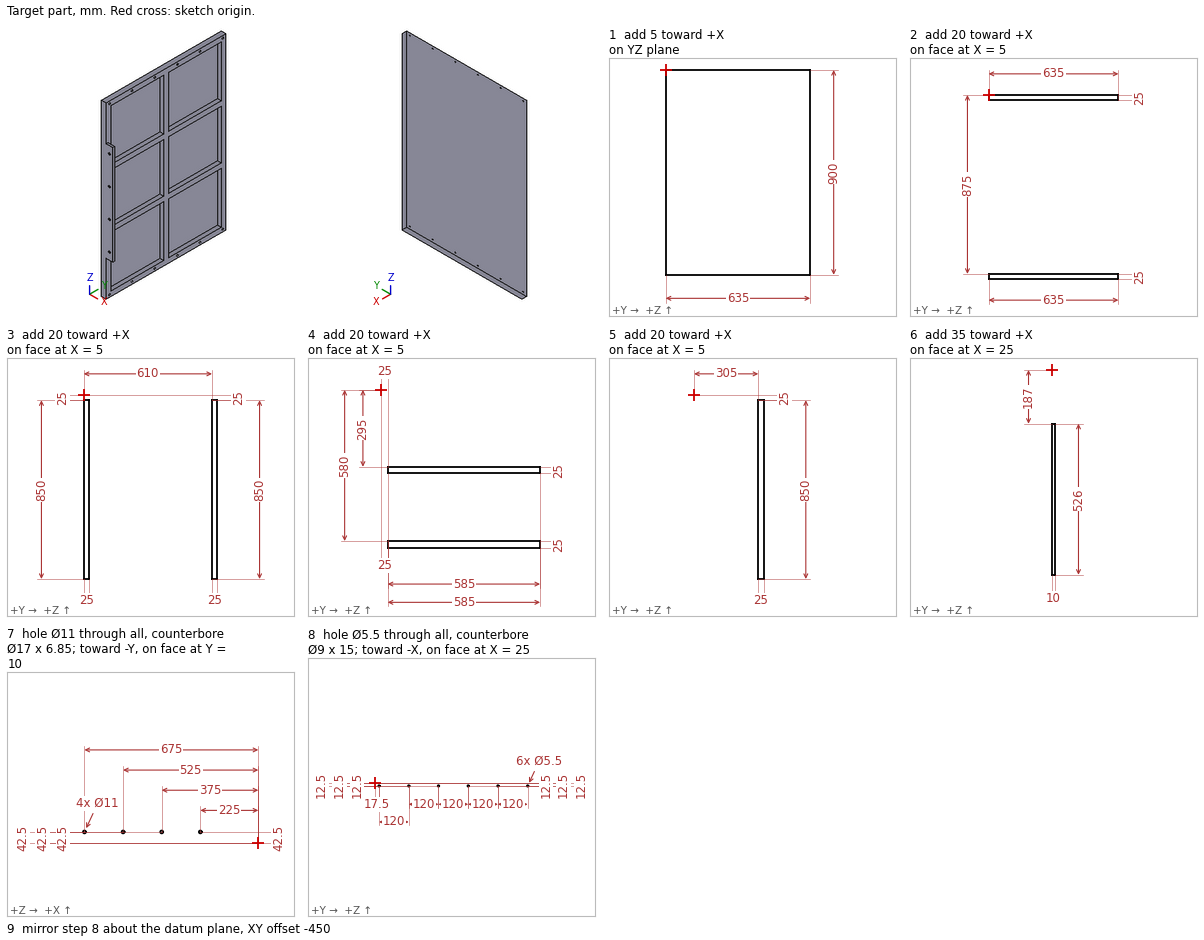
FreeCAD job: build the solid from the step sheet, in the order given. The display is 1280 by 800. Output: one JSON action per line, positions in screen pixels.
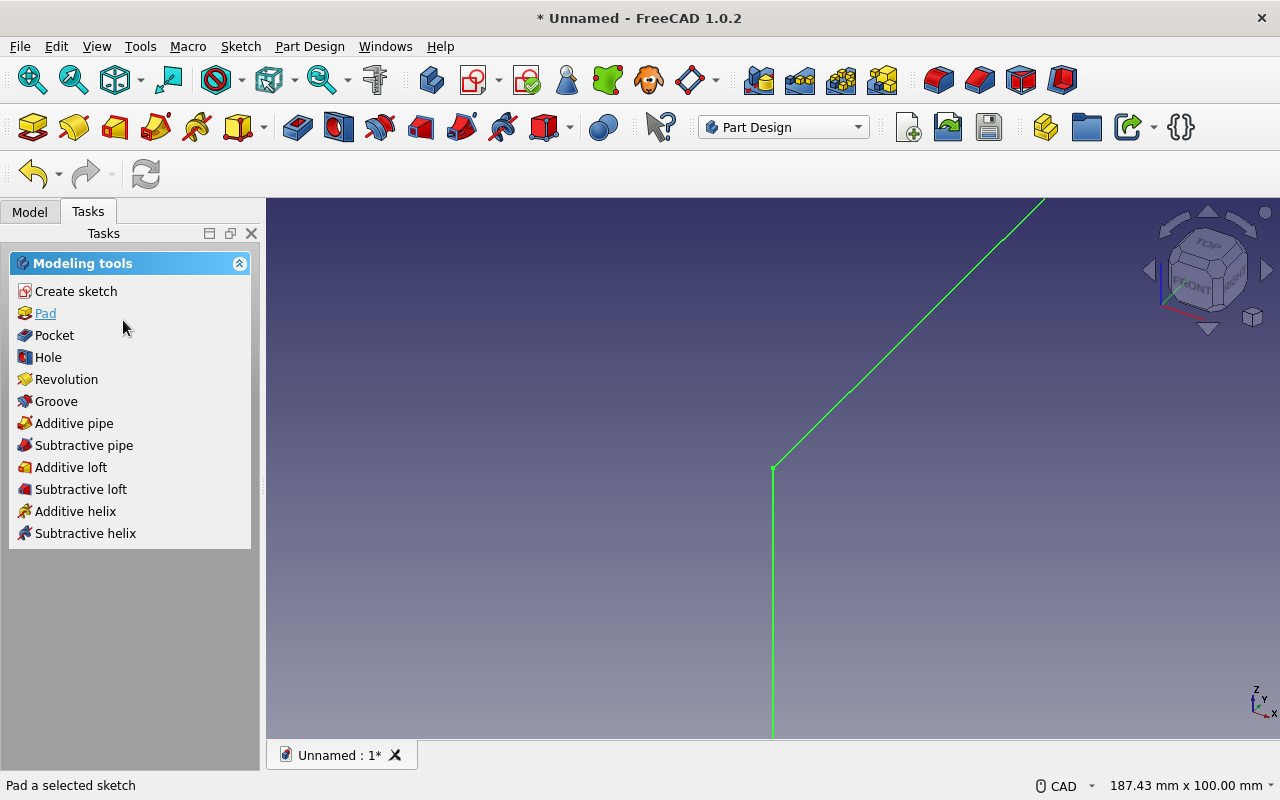
{"action": "left_click", "coordinate": [33, 128]}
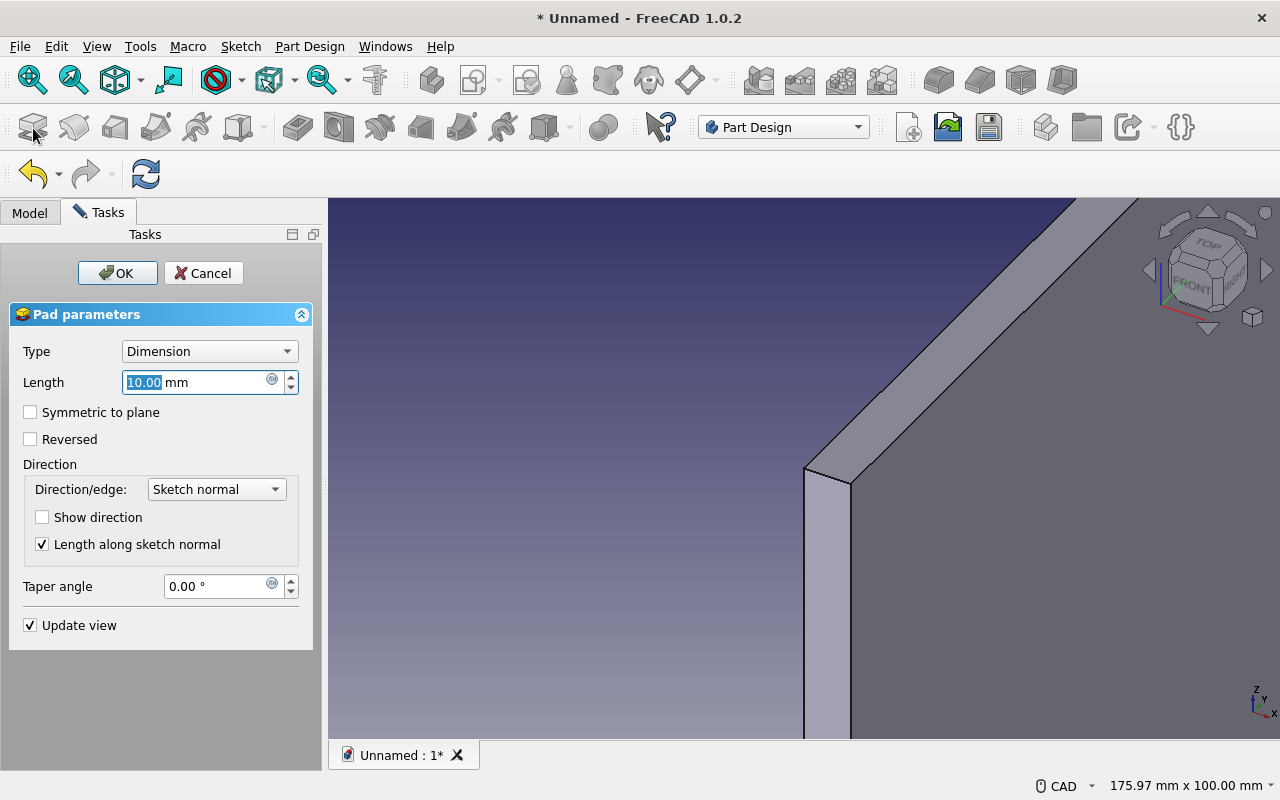
{"action": "type", "text": "5"}
{"action": "key", "text": "Tab"}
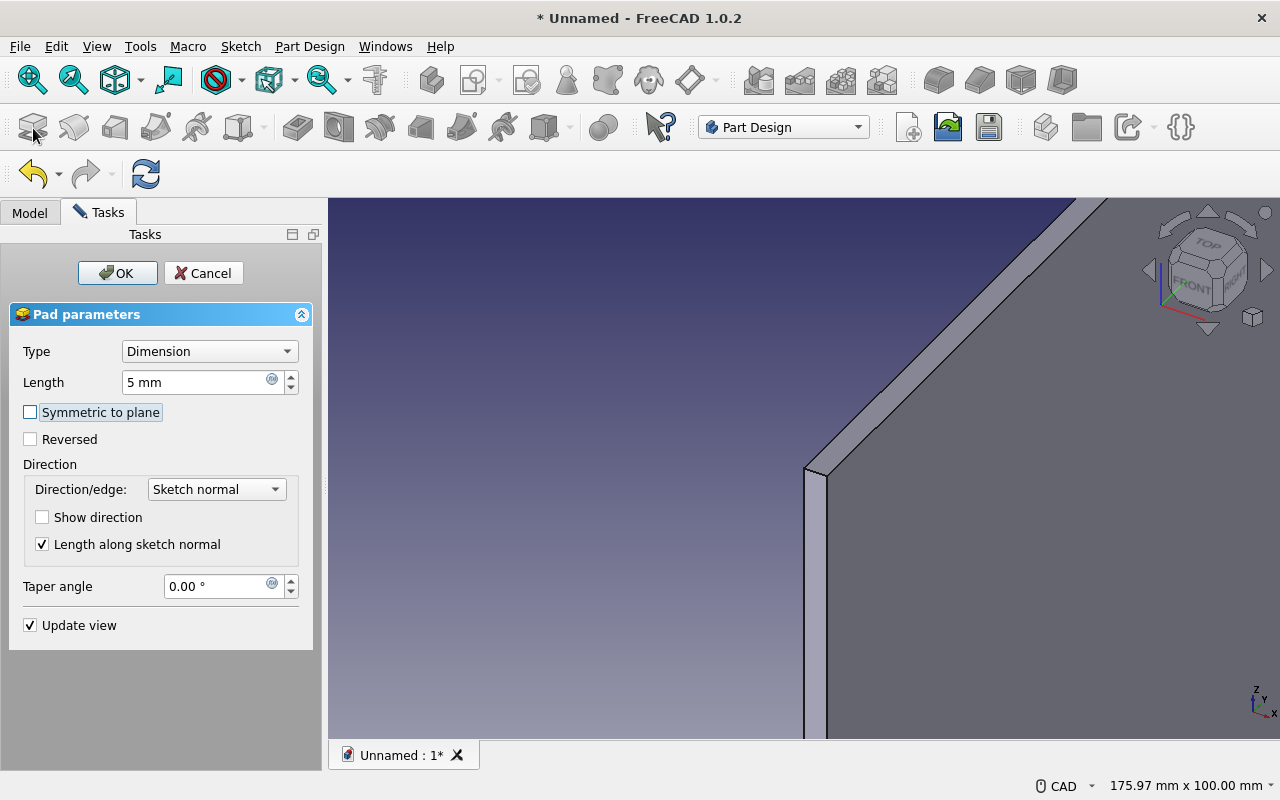
{"action": "left_click", "coordinate": [118, 273]}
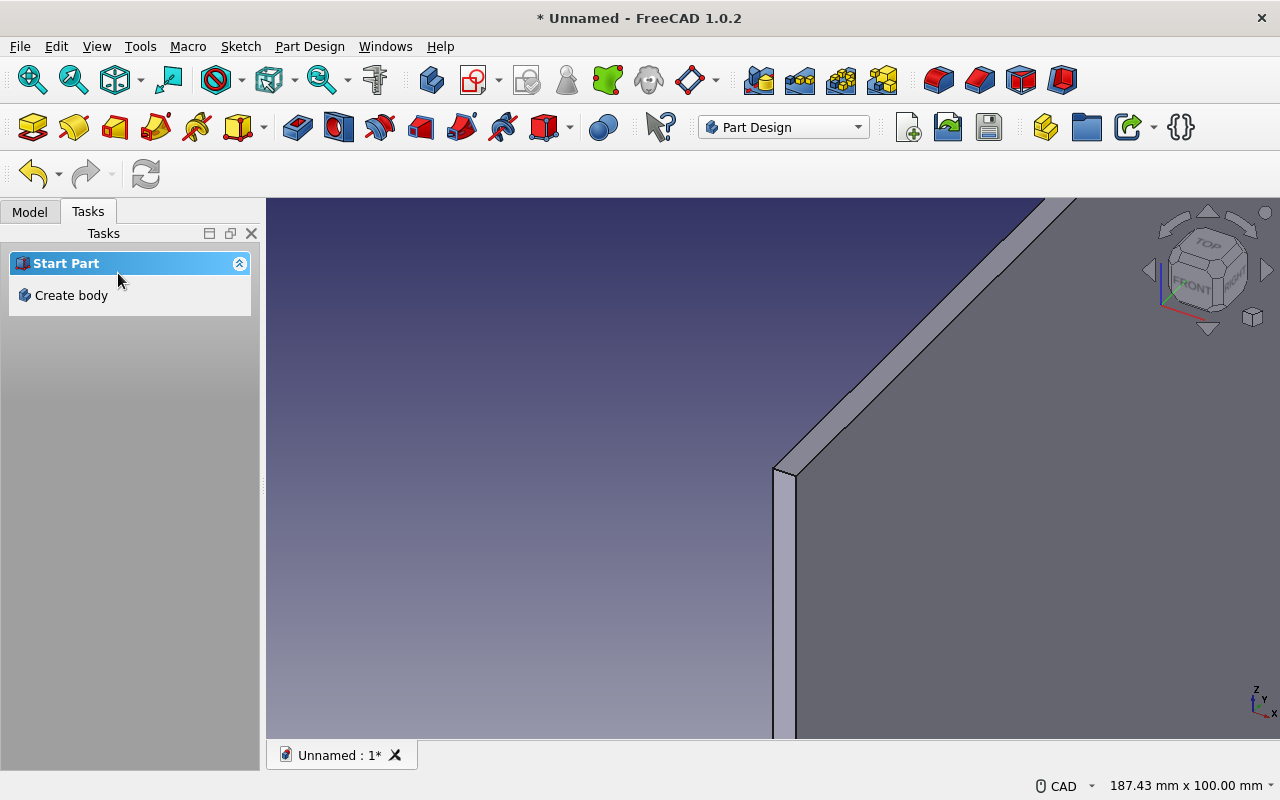
{"action": "left_click", "coordinate": [33, 80]}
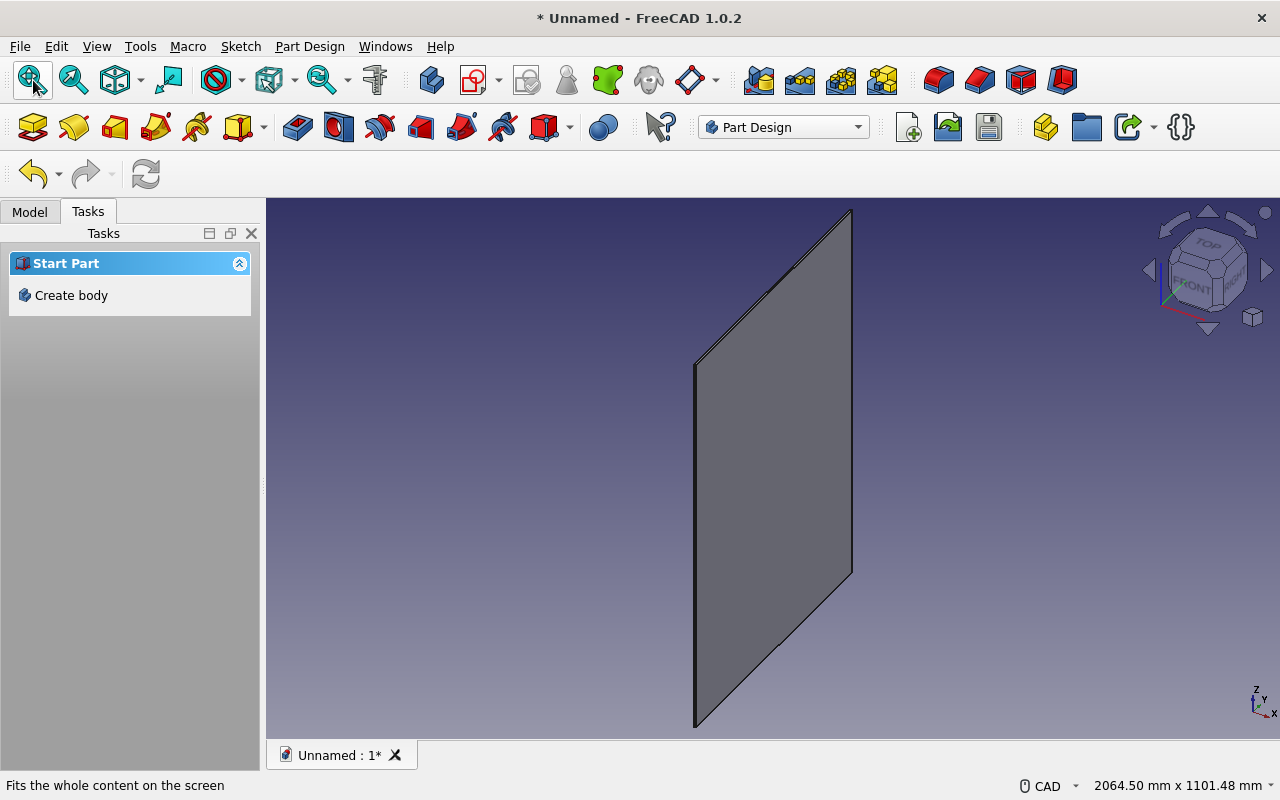
{"action": "left_click", "coordinate": [774, 416]}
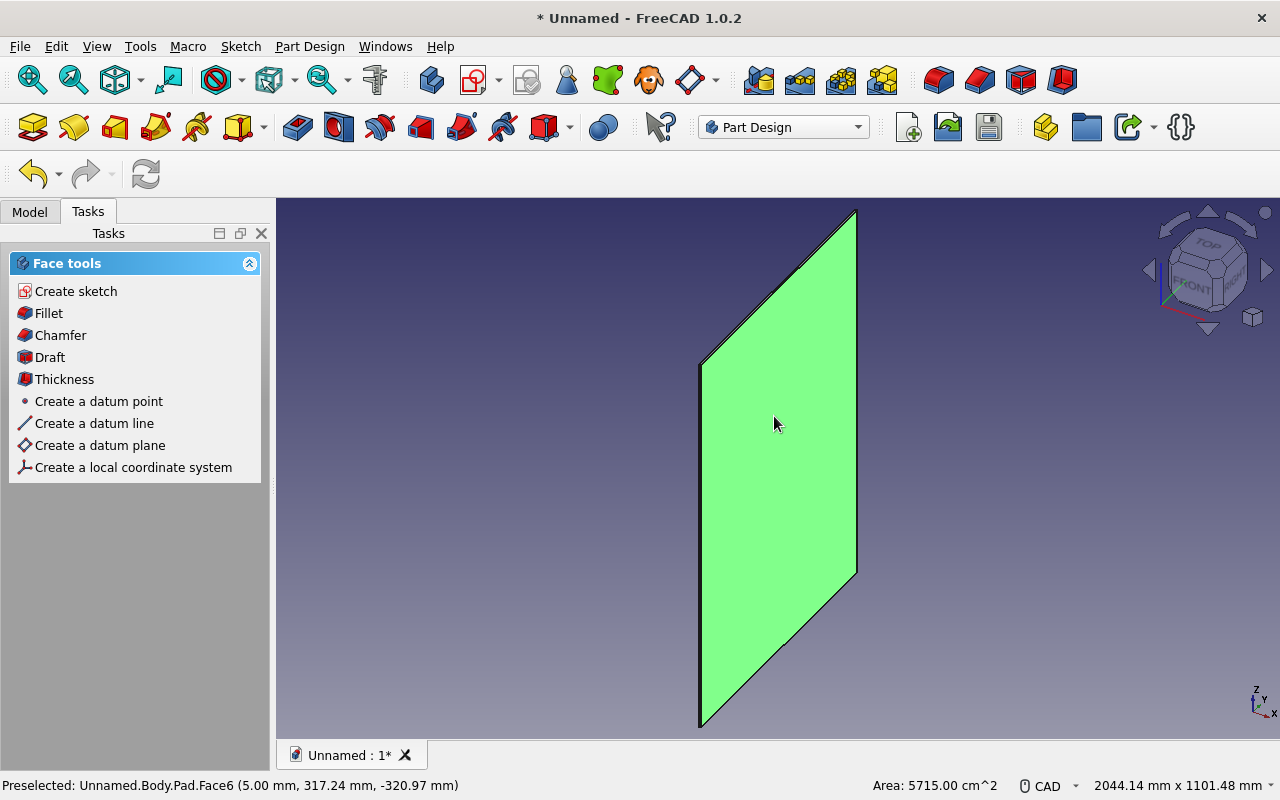
{"action": "left_click", "coordinate": [472, 80]}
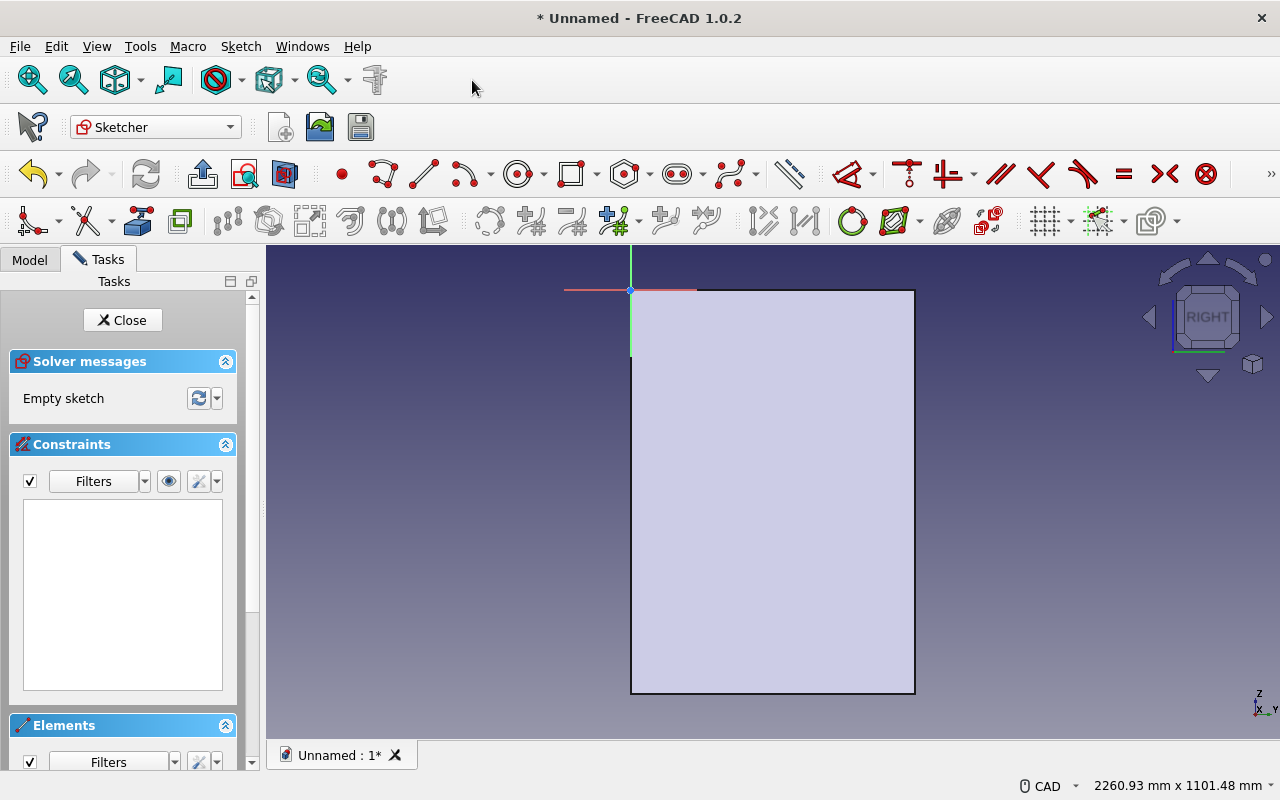
{"action": "scroll", "coordinate": [395, 492], "scroll_direction": "down", "scroll_amount": 1}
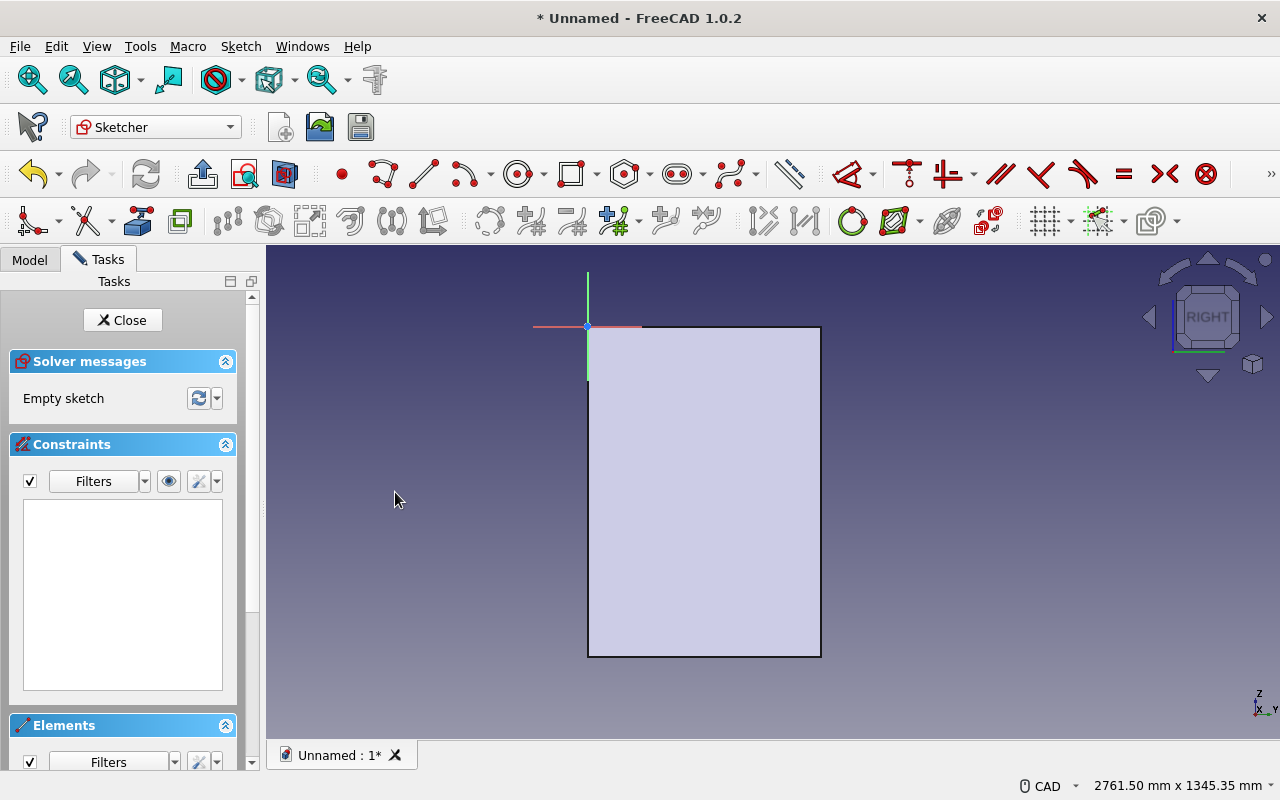
{"action": "left_click", "coordinate": [570, 174]}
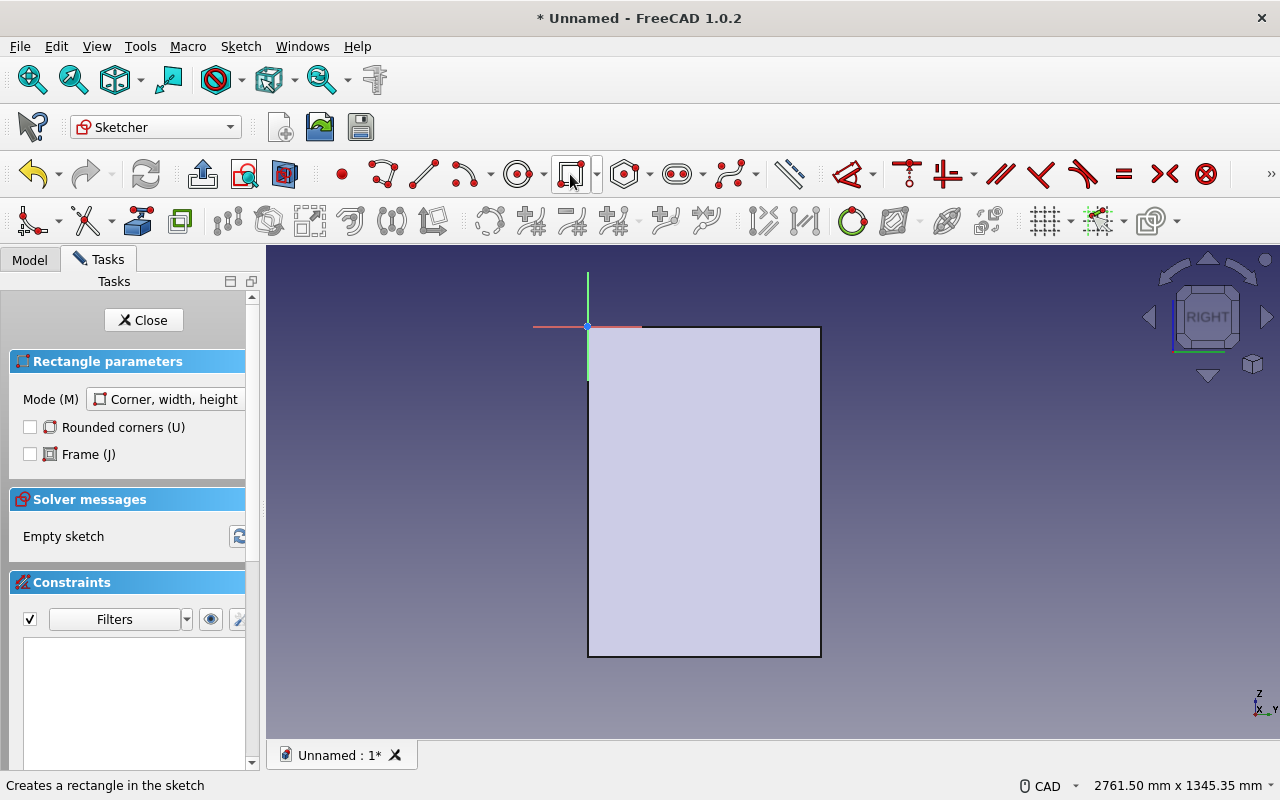
{"action": "scroll", "coordinate": [588, 327], "scroll_direction": "up", "scroll_amount": 3}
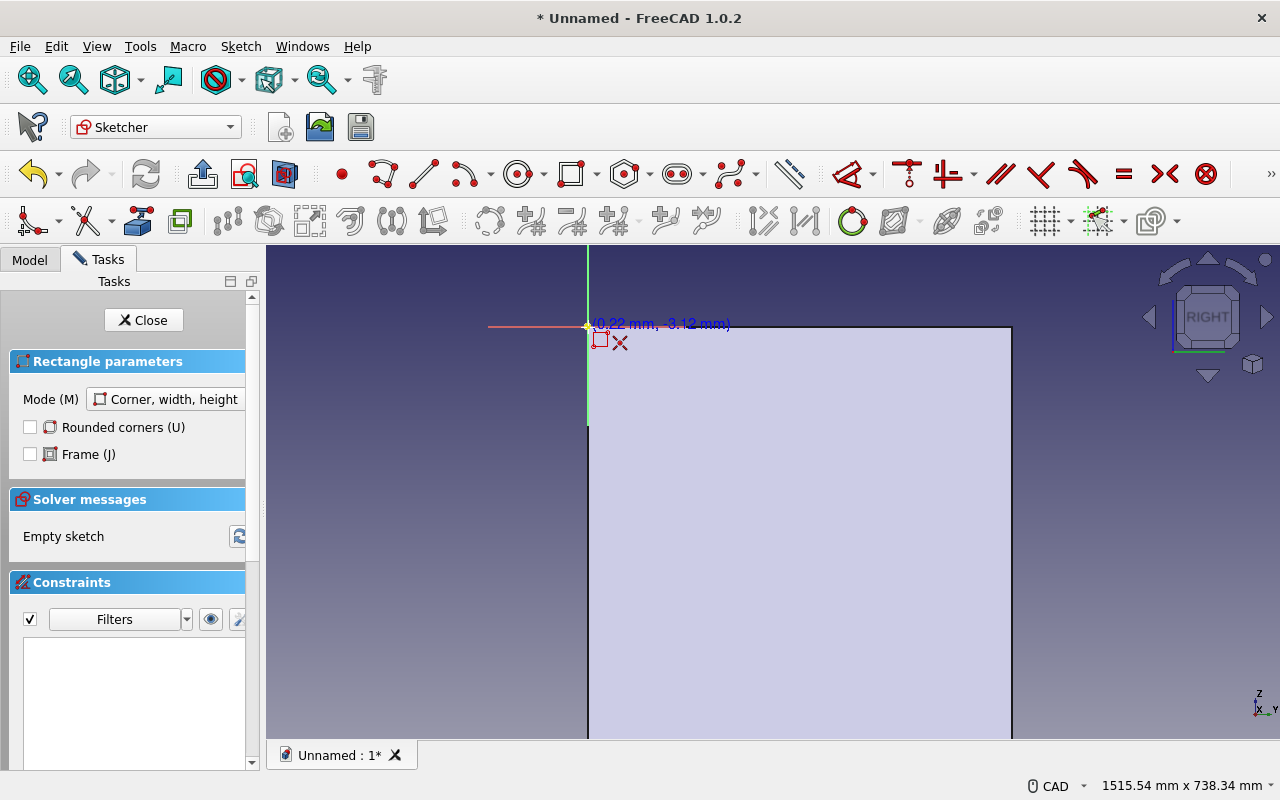
{"action": "left_click", "coordinate": [588, 327]}
{"action": "mouse_move", "coordinate": [1012, 343]}